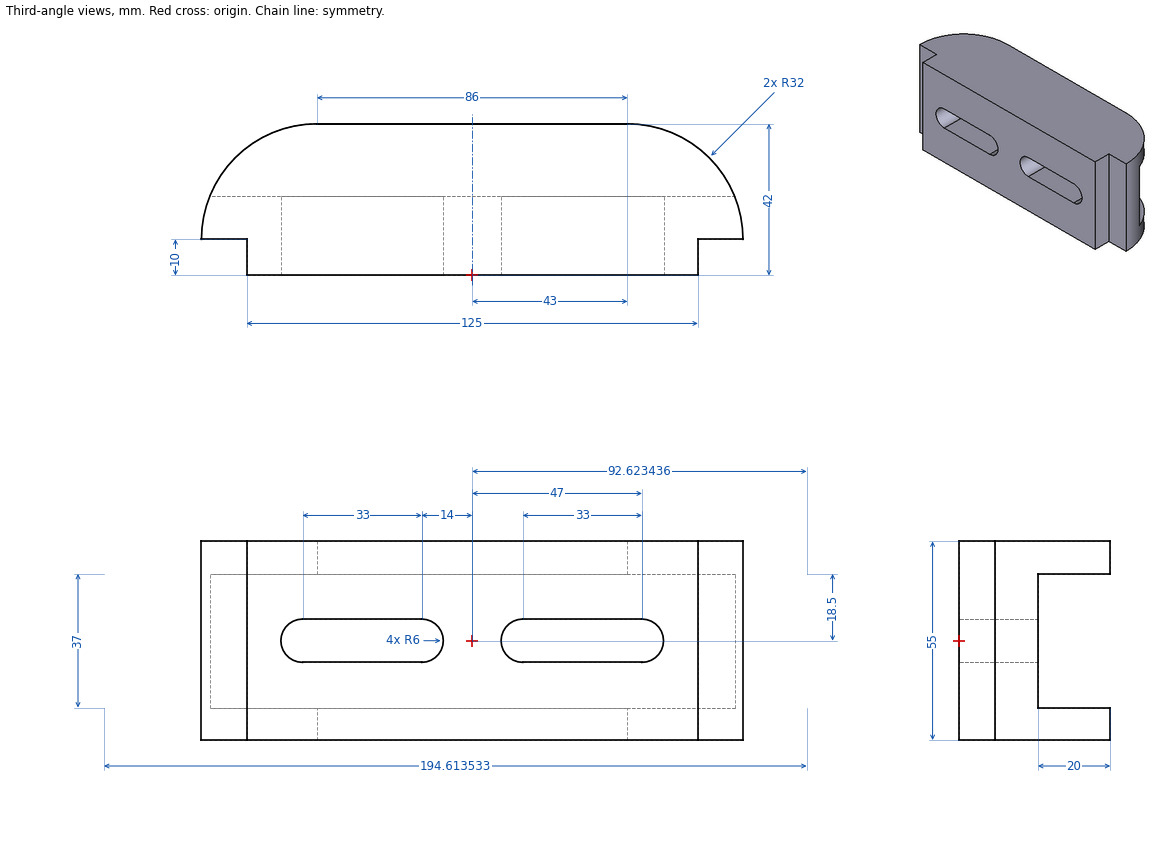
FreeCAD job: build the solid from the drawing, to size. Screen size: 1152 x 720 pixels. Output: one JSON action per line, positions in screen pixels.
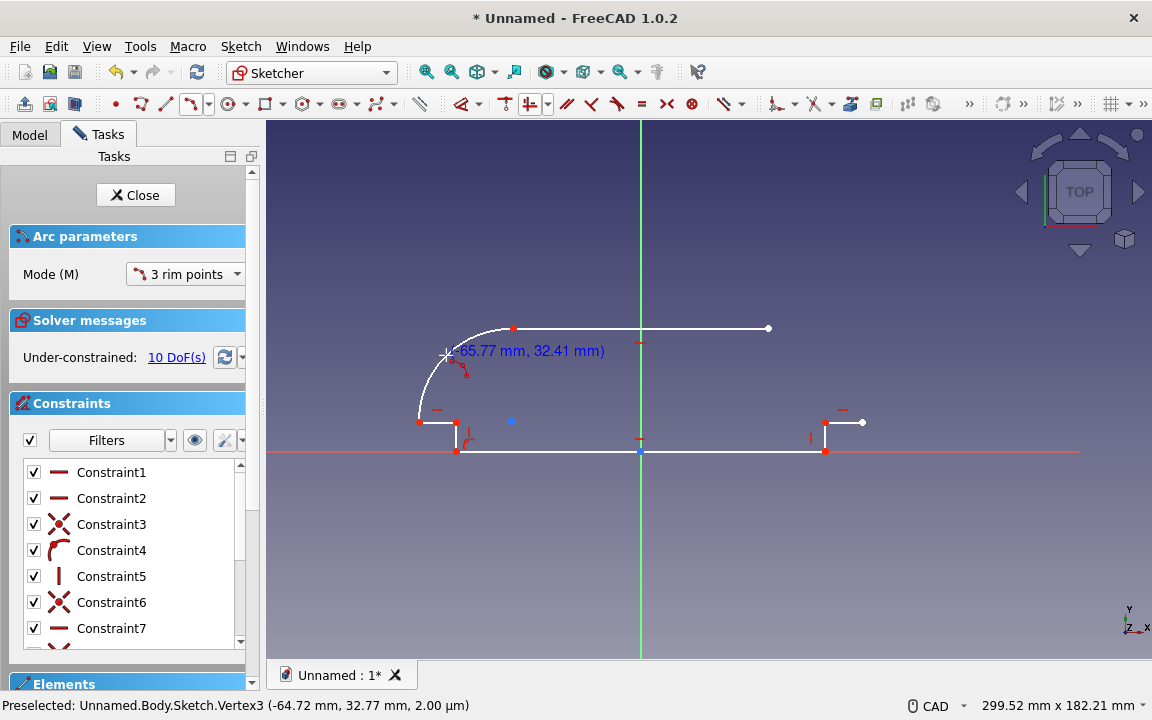
{"action": "left_click", "coordinate": [862, 423]}
{"action": "left_click", "coordinate": [768, 329]}
{"action": "left_click", "coordinate": [835, 355]}
{"action": "key", "text": "Escape"}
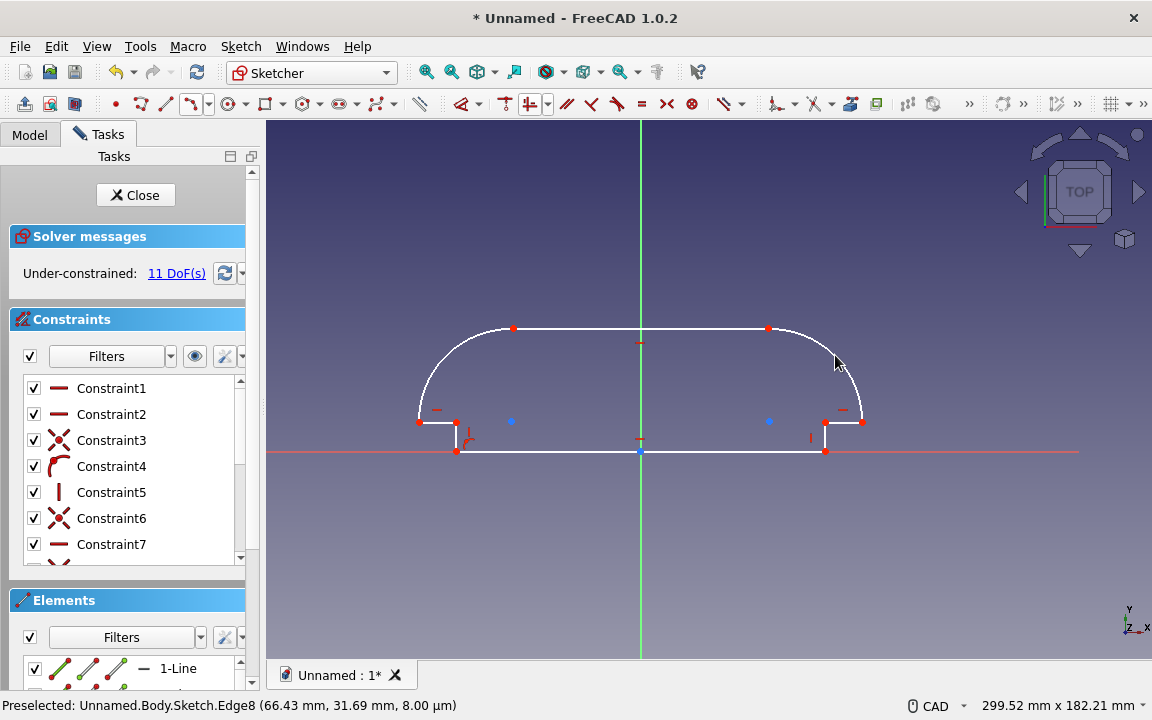
{"action": "left_click", "coordinate": [692, 329]}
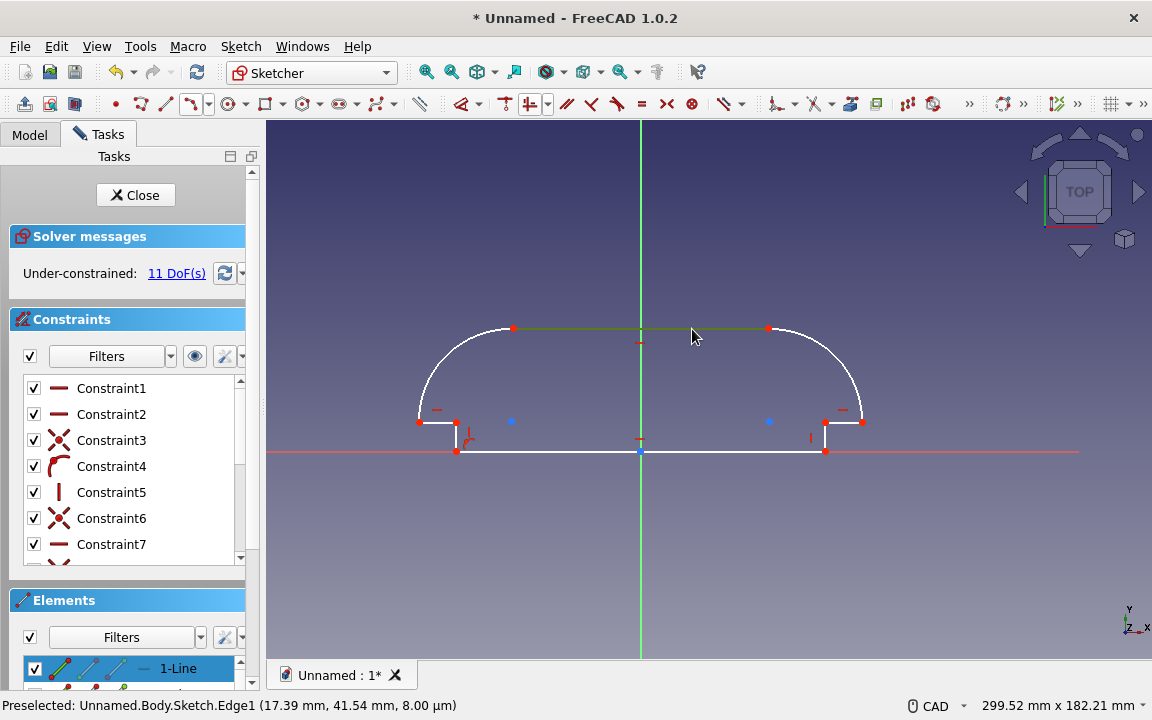
{"action": "left_click", "coordinate": [470, 339]}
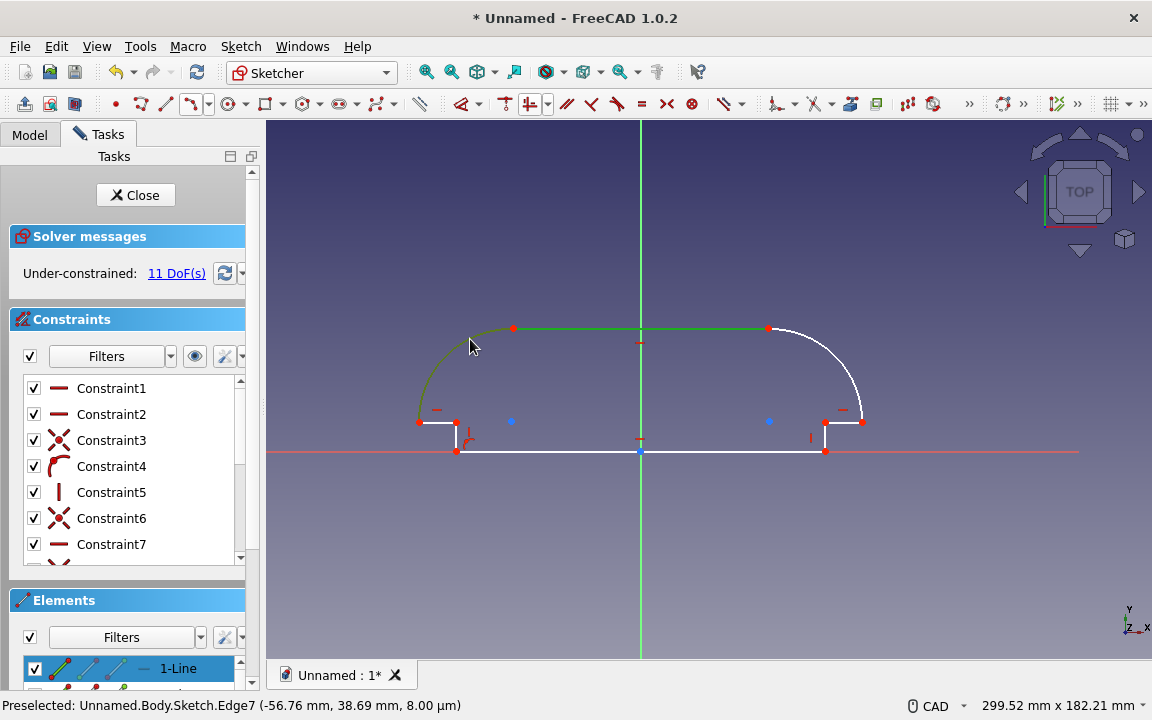
{"action": "left_click", "coordinate": [617, 104]}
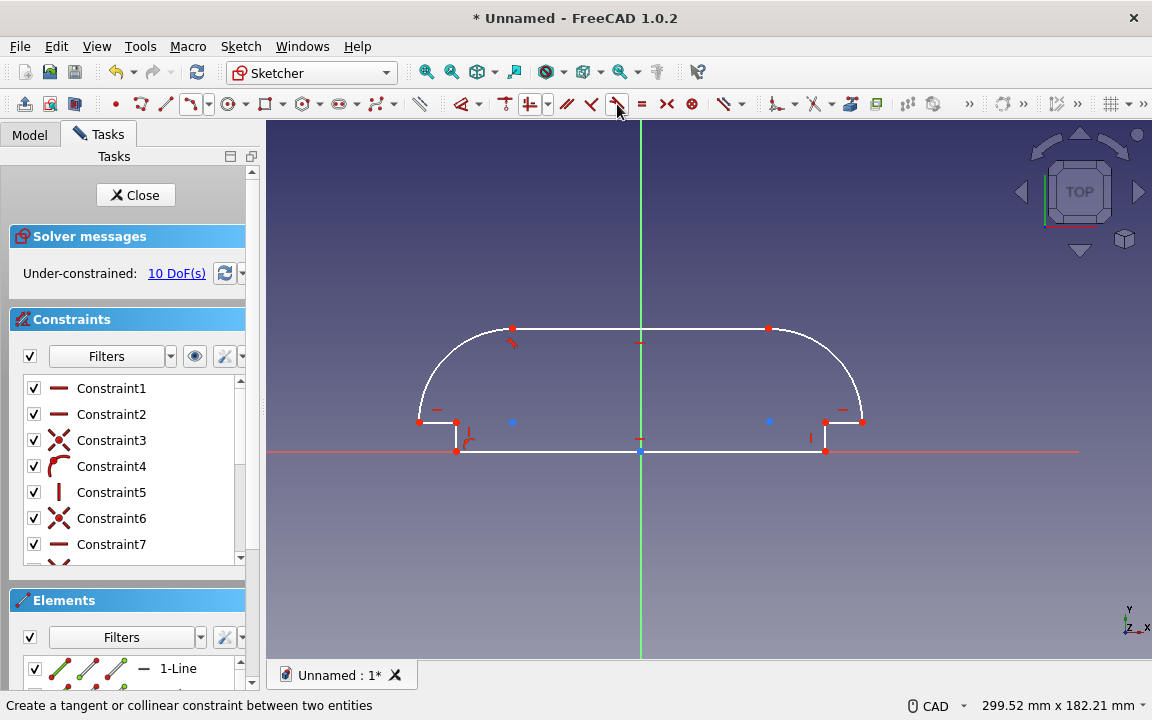
{"action": "left_click", "coordinate": [691, 329]}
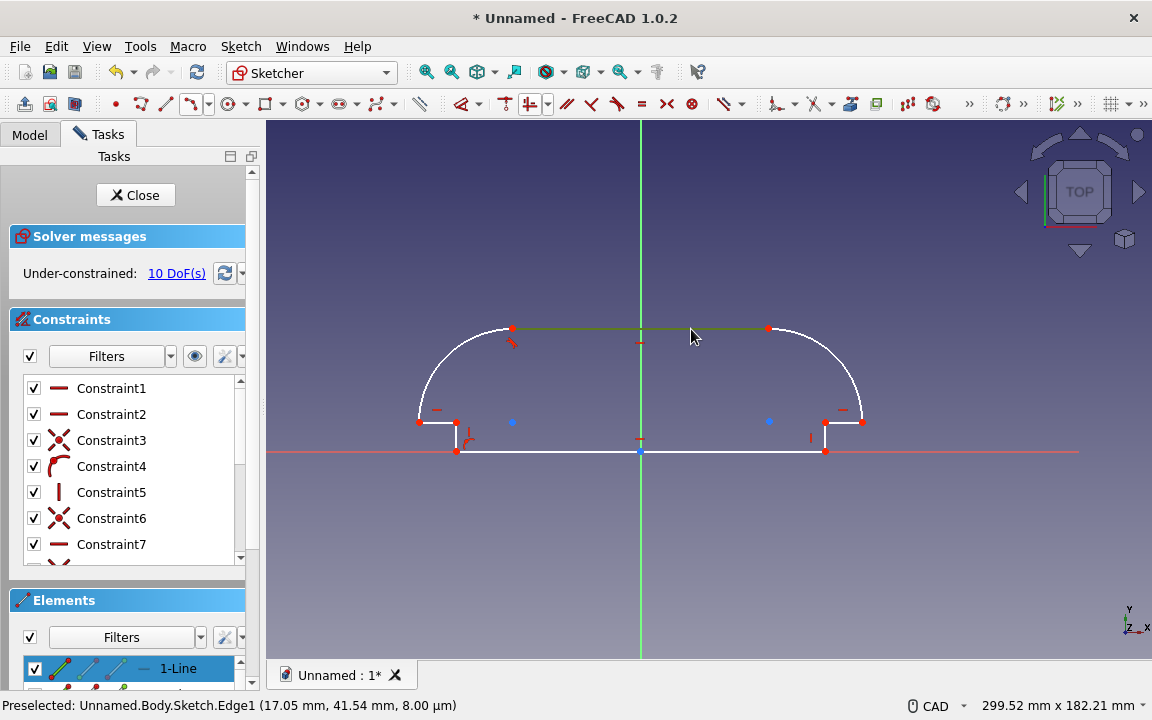
{"action": "left_click", "coordinate": [852, 380]}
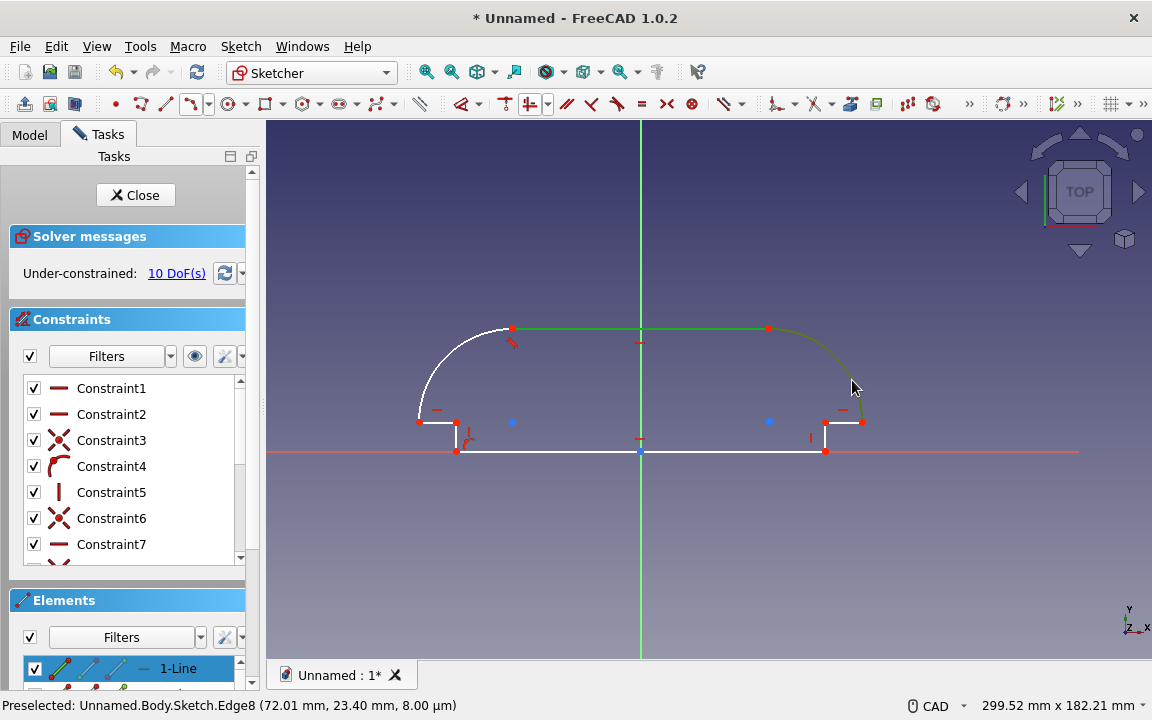
{"action": "left_click", "coordinate": [617, 104]}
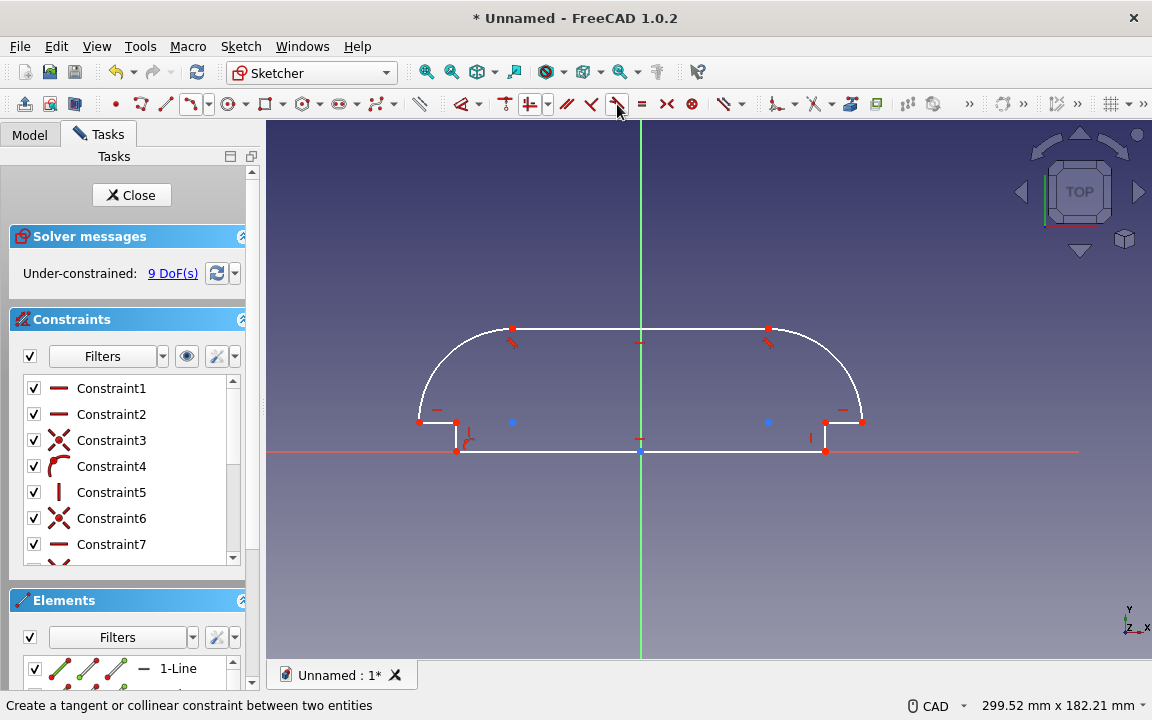
{"action": "left_click", "coordinate": [470, 339]}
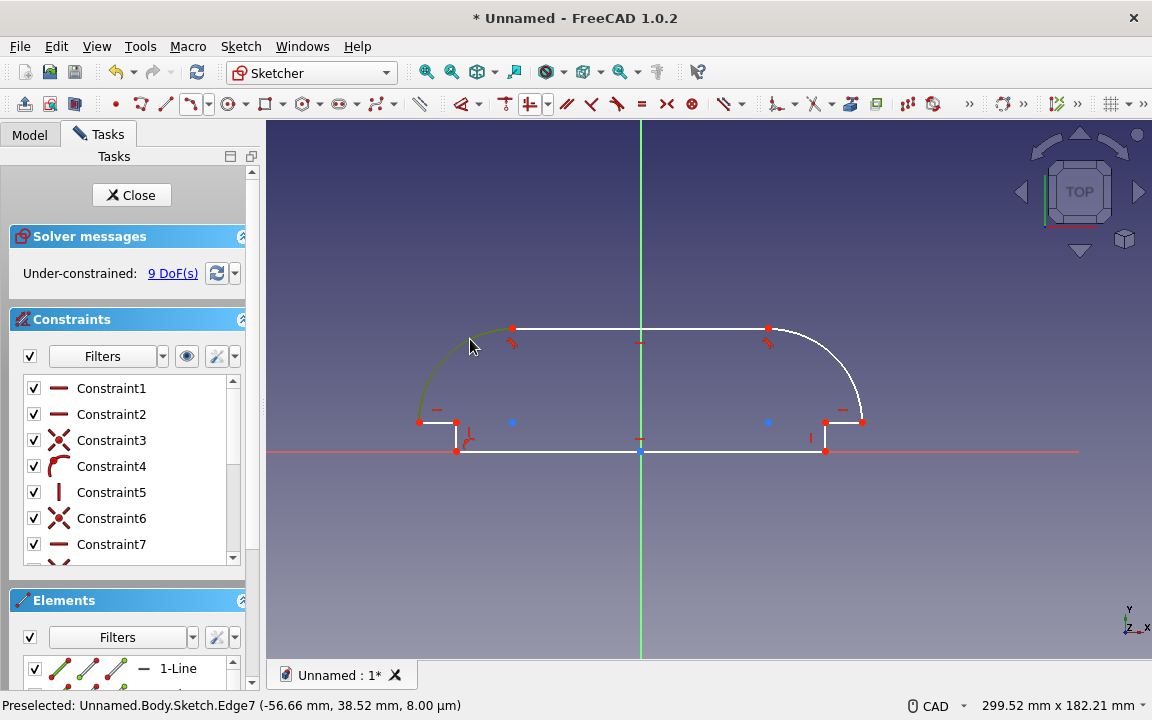
{"action": "left_click", "coordinate": [852, 380]}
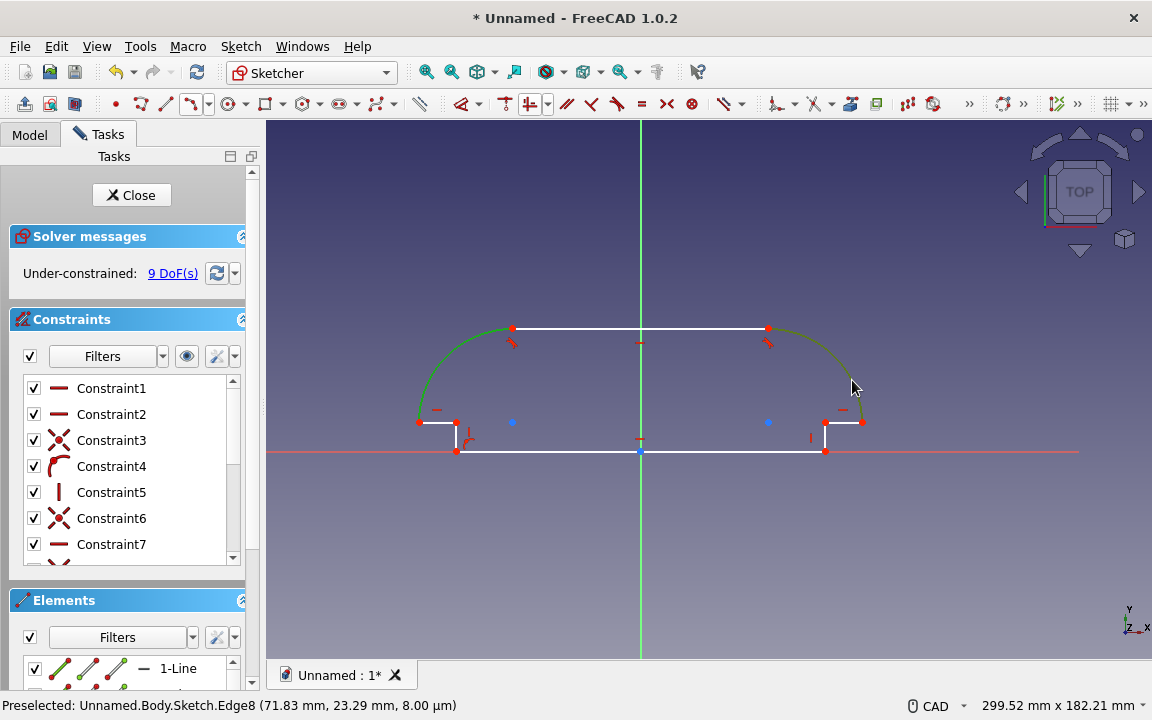
{"action": "left_click", "coordinate": [642, 104]}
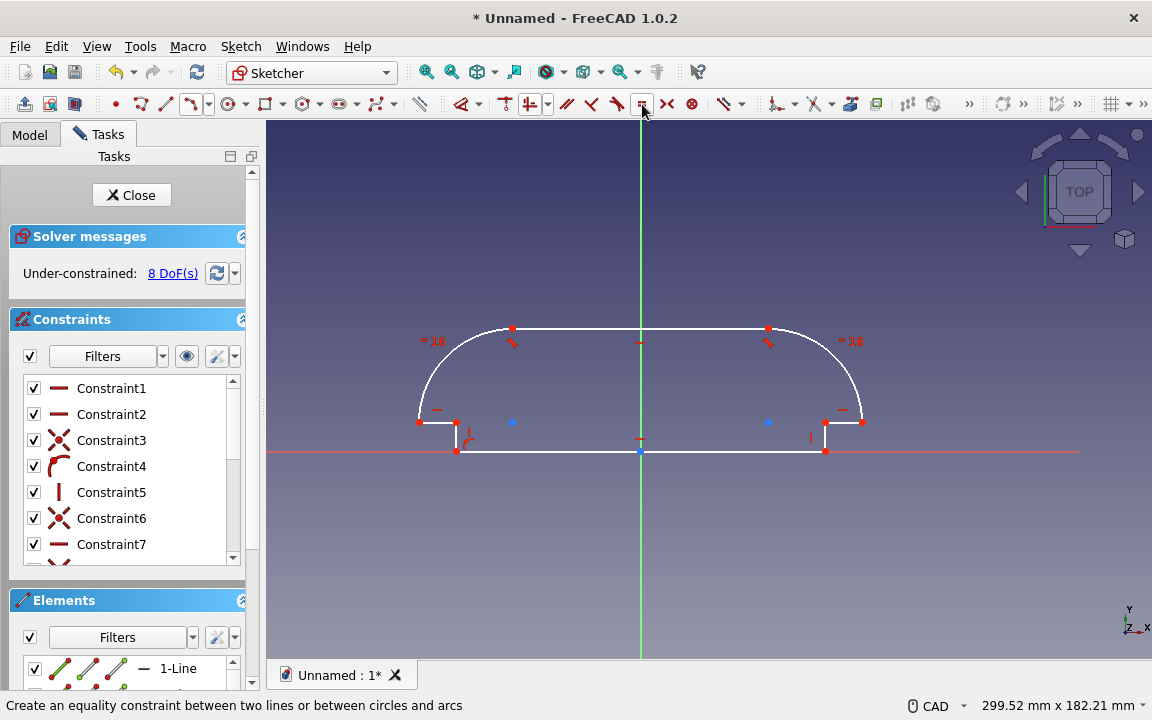
{"action": "left_click", "coordinate": [456, 423]}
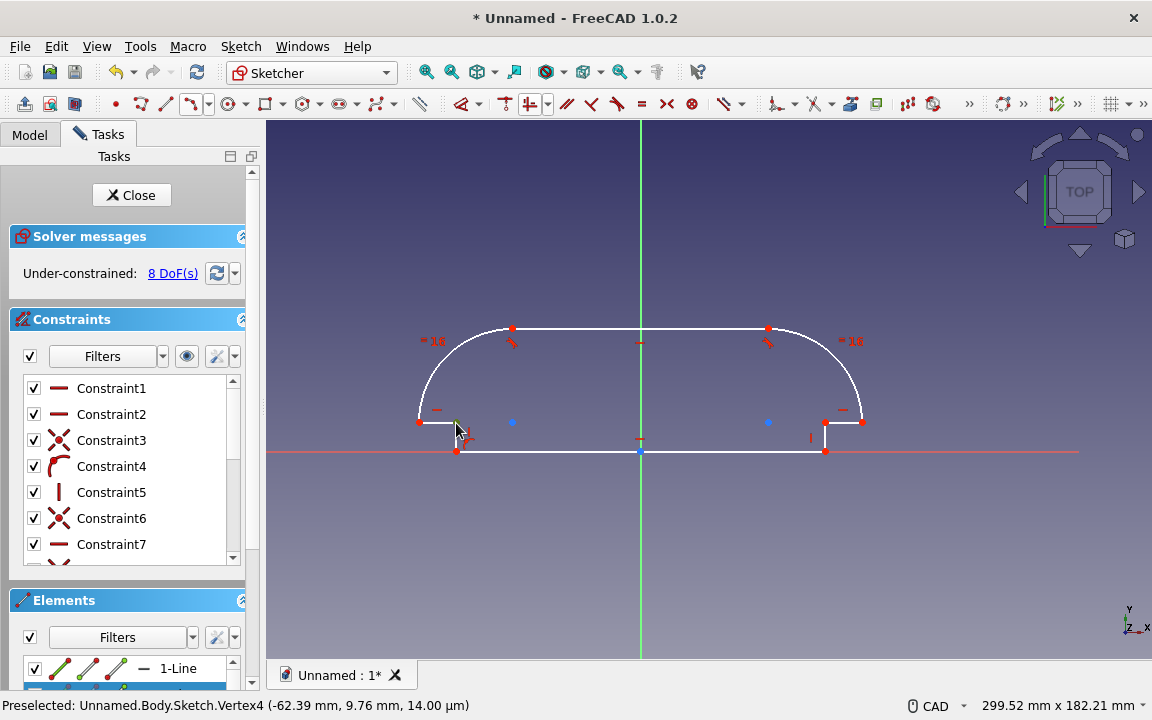
{"action": "left_click", "coordinate": [825, 423]}